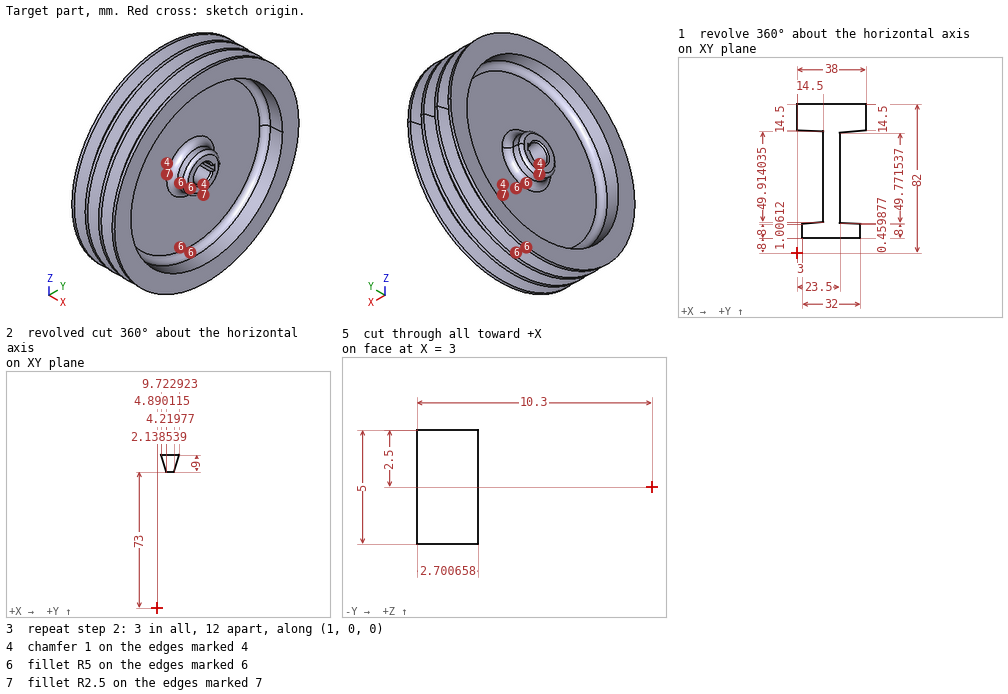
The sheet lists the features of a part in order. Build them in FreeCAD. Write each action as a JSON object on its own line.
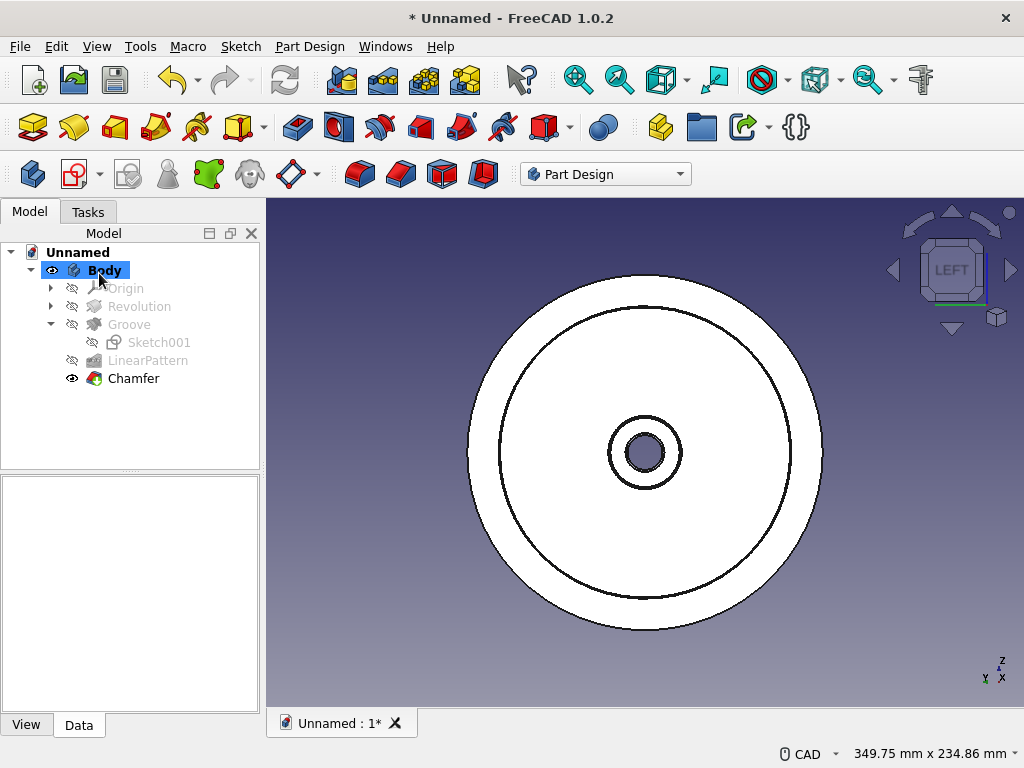
{"action": "scroll", "coordinate": [665, 471], "scroll_direction": "up", "scroll_amount": 3}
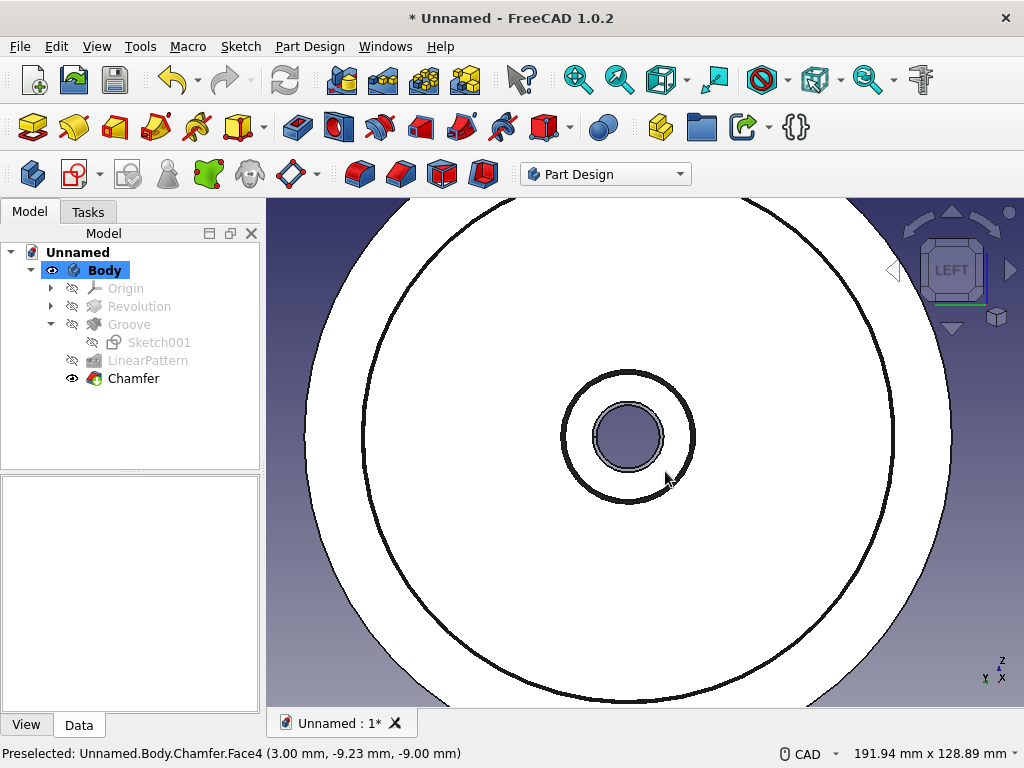
{"action": "left_click", "coordinate": [664, 472]}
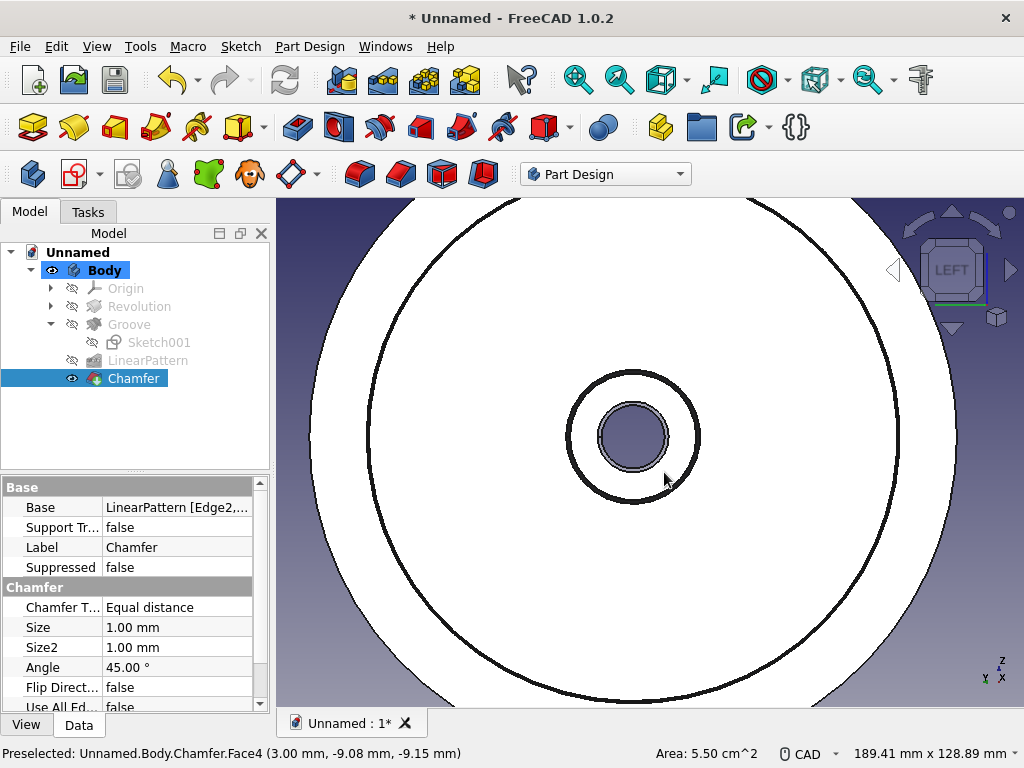
{"action": "left_click", "coordinate": [74, 174]}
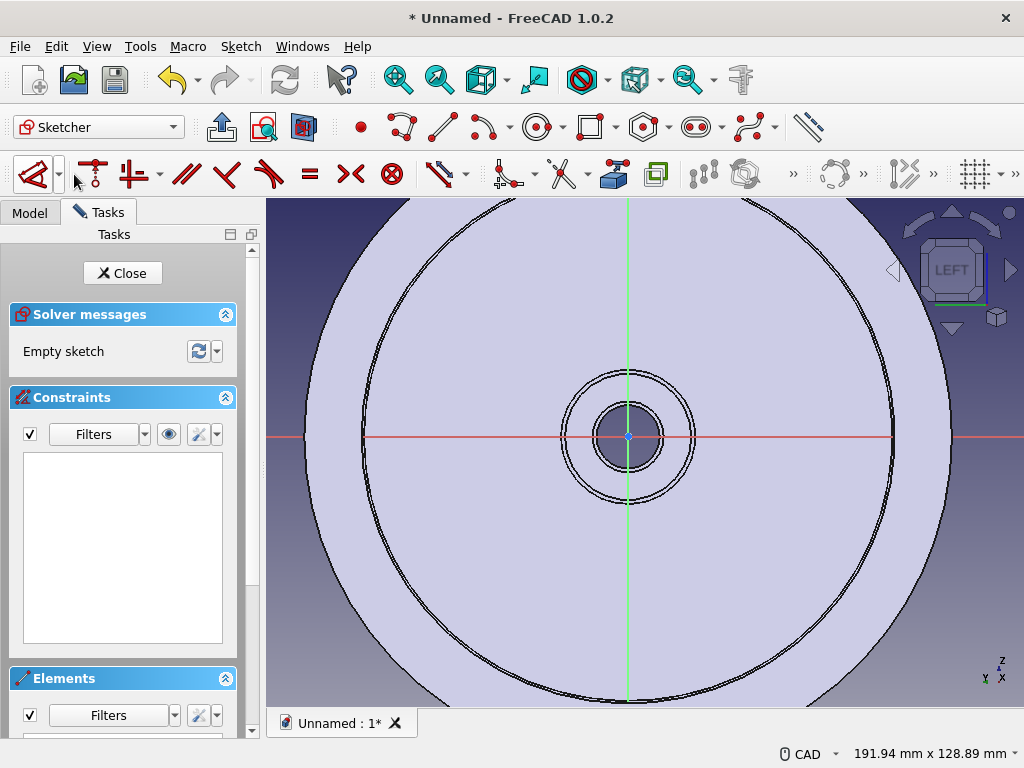
{"action": "left_click", "coordinate": [304, 128]}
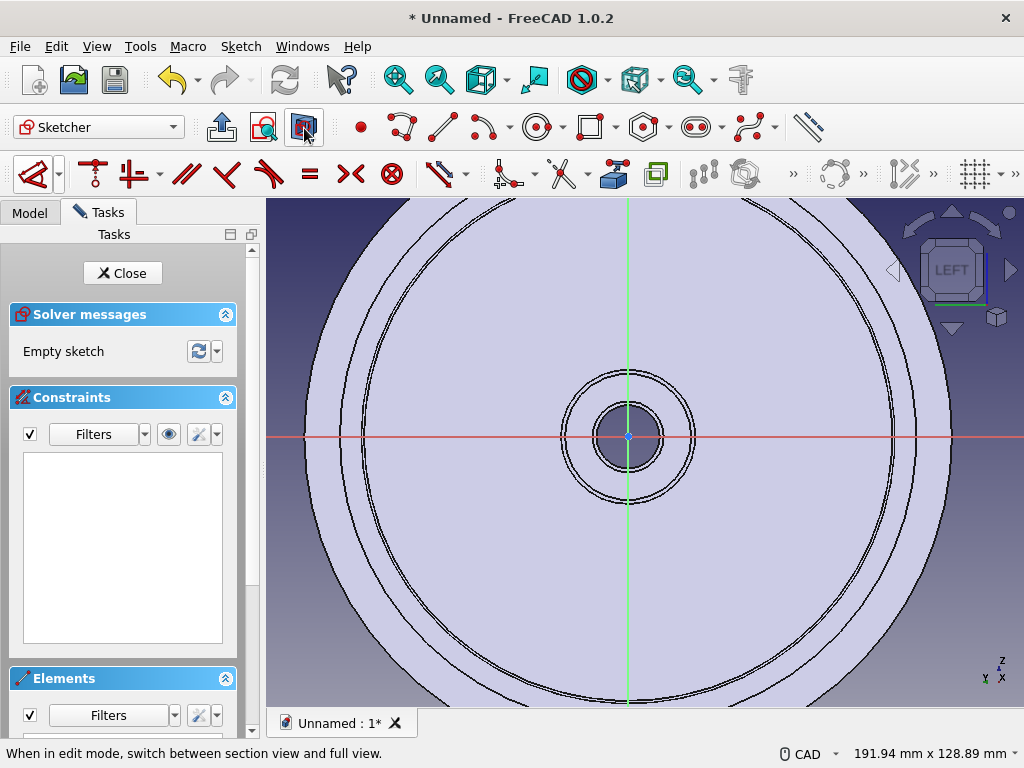
{"action": "scroll", "coordinate": [612, 435], "scroll_direction": "up", "scroll_amount": 11}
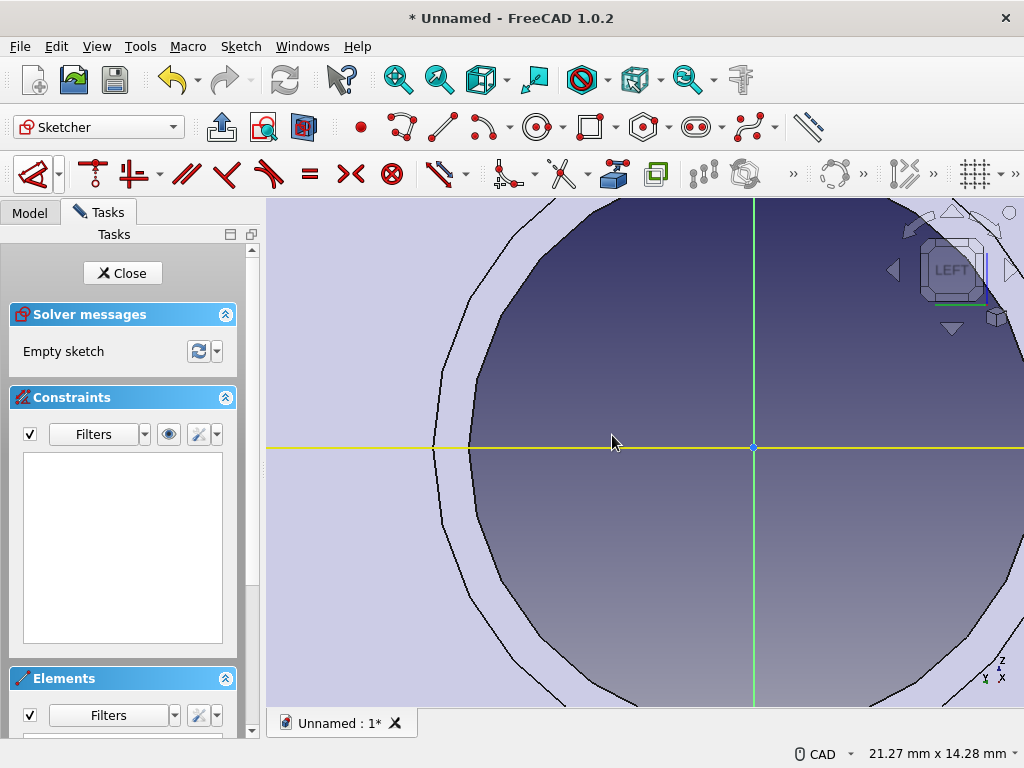
{"action": "left_click", "coordinate": [590, 128]}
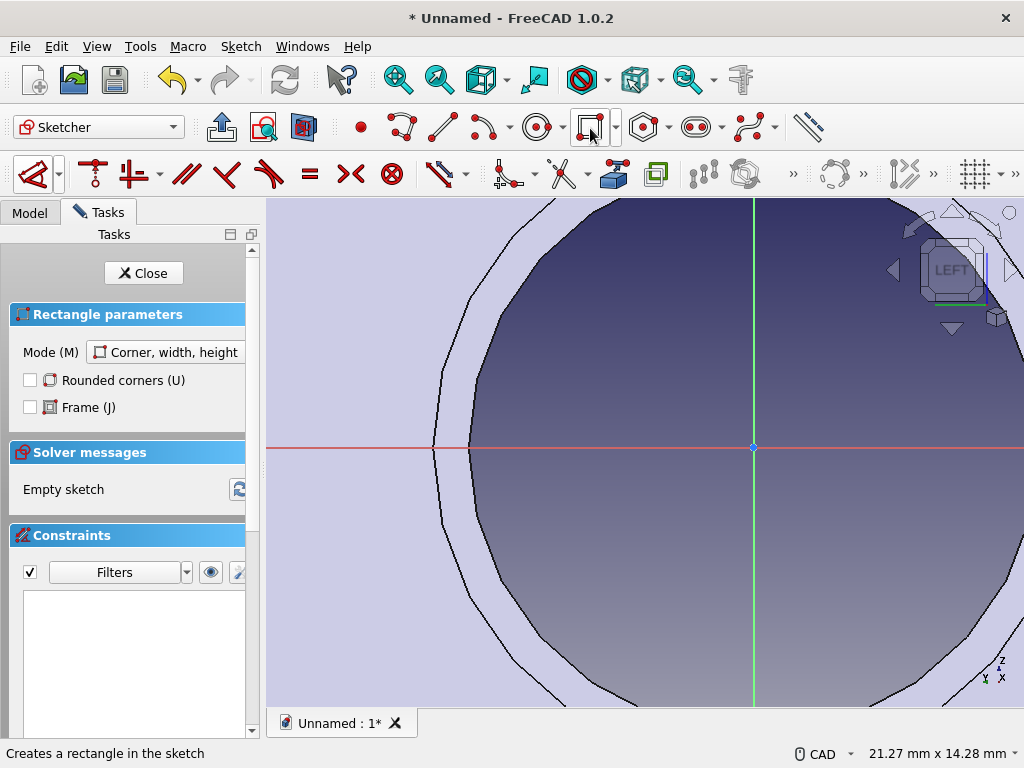
{"action": "left_click", "coordinate": [387, 359]}
{"action": "left_click", "coordinate": [483, 537]}
{"action": "key", "text": "Escape"}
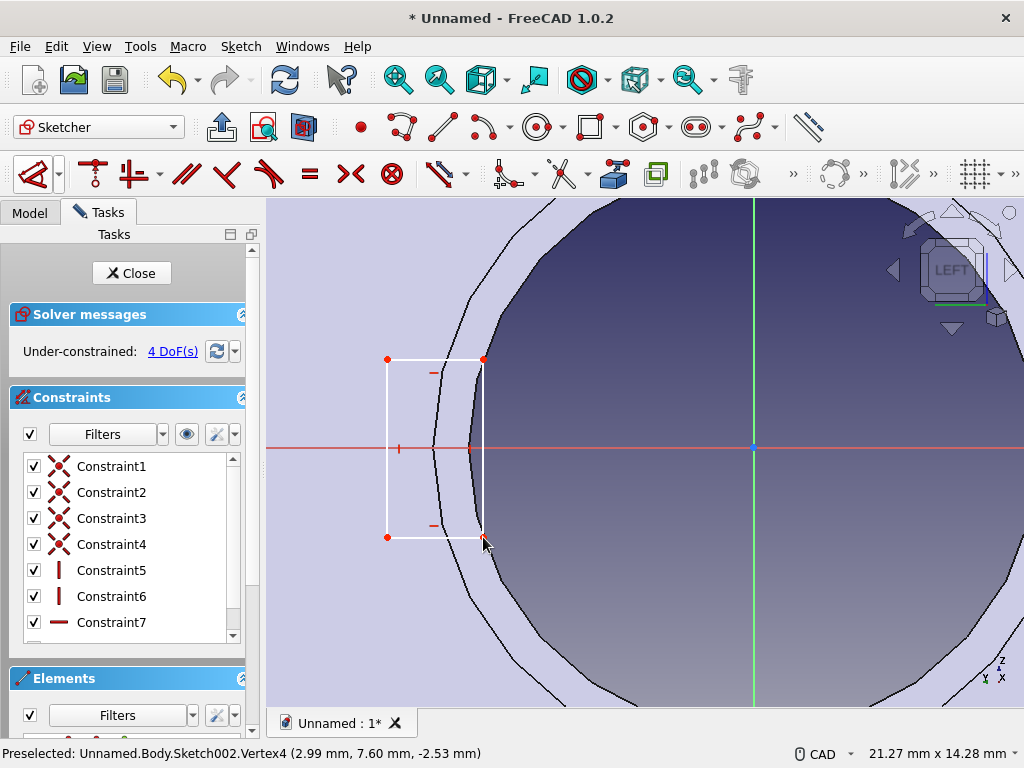
{"action": "left_click", "coordinate": [387, 413]}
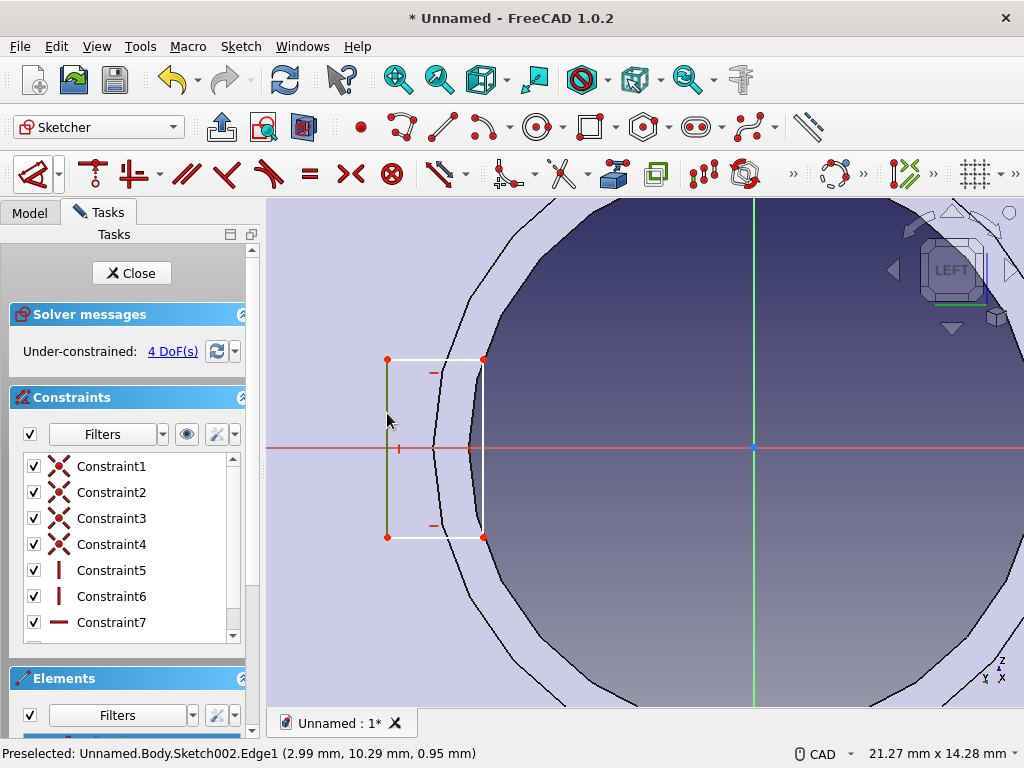
{"action": "left_click", "coordinate": [58, 174]}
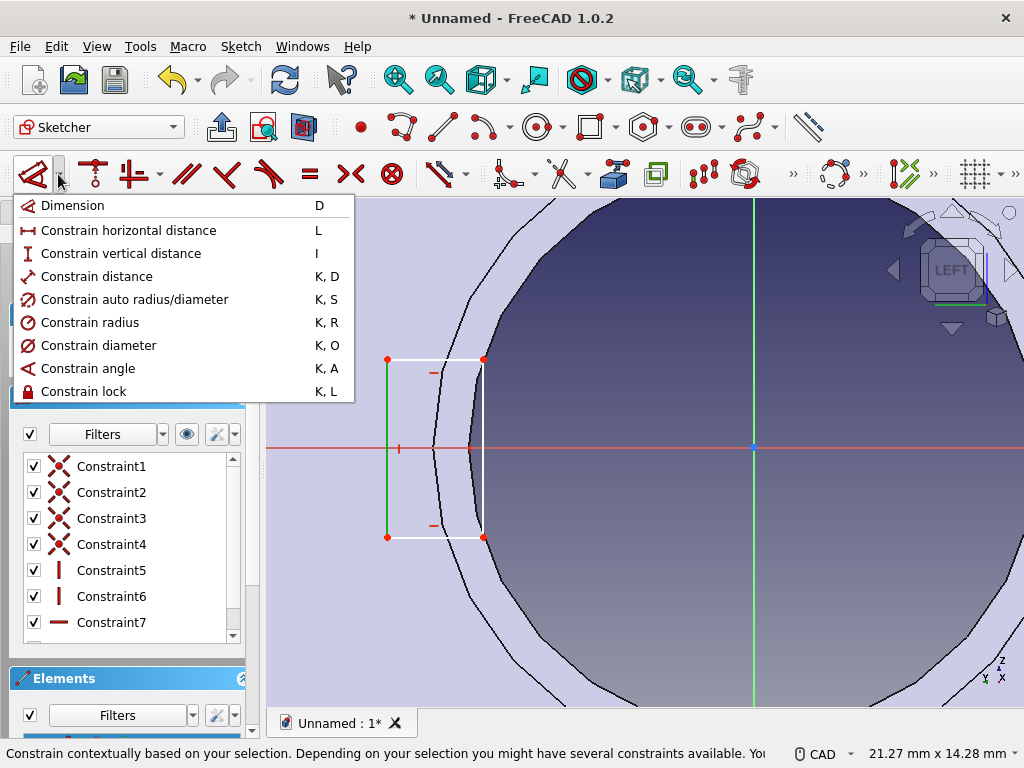
{"action": "left_click", "coordinate": [184, 254]}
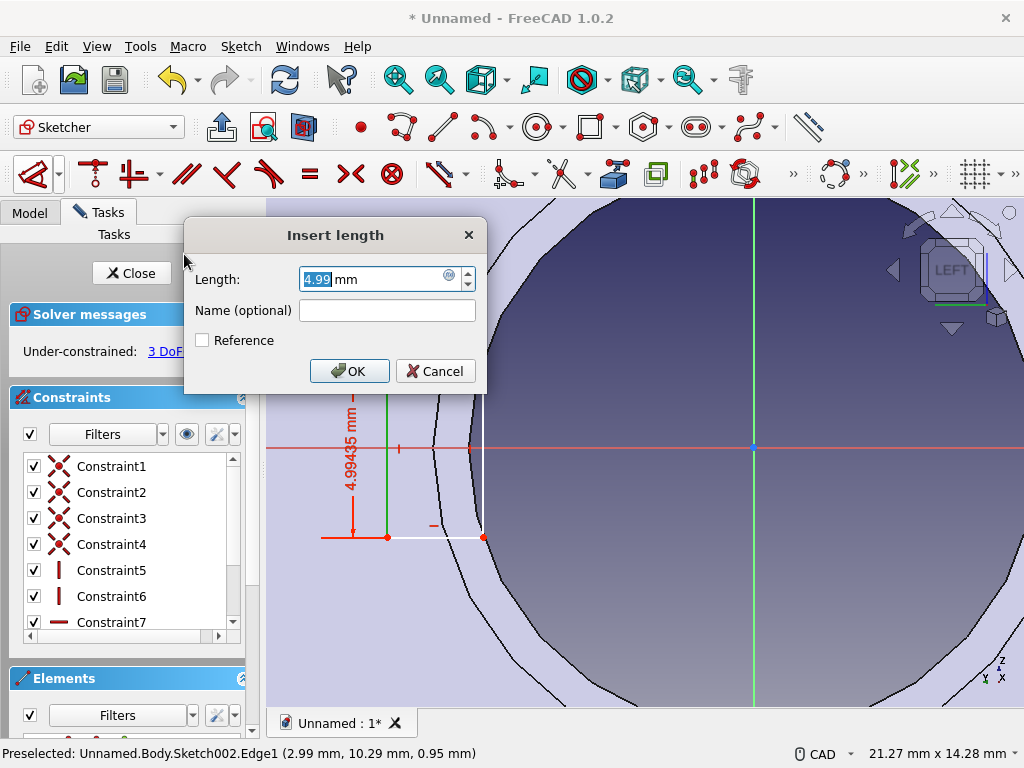
{"action": "type", "text": "5"}
{"action": "key", "text": "Return"}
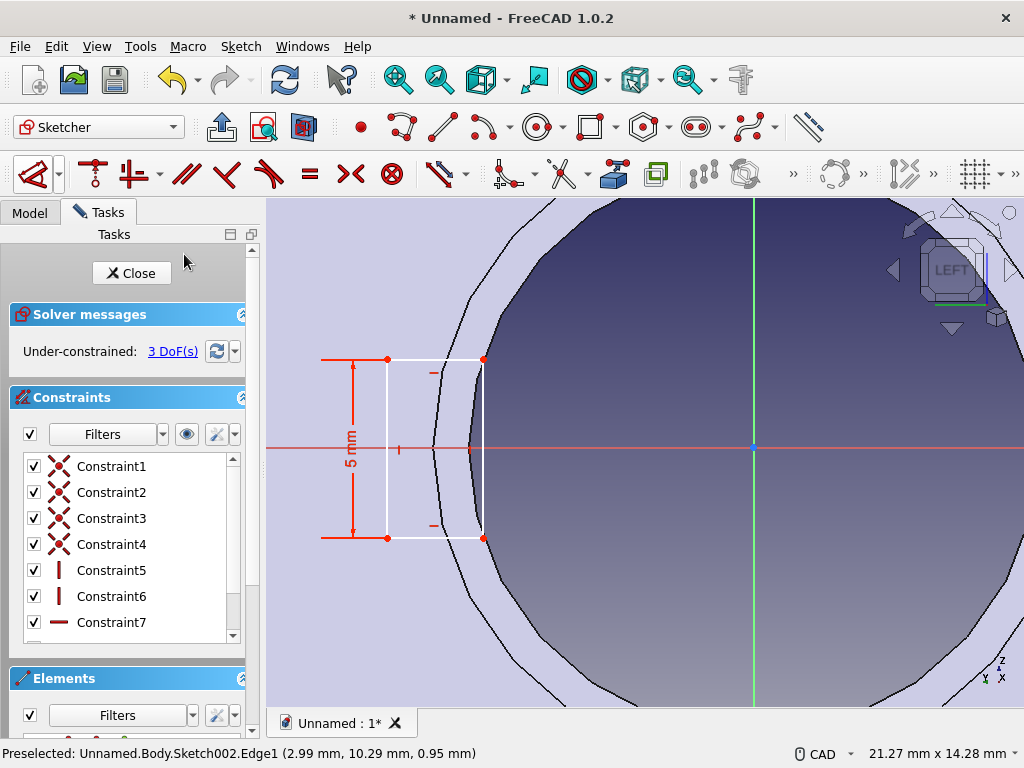
{"action": "left_click", "coordinate": [387, 360]}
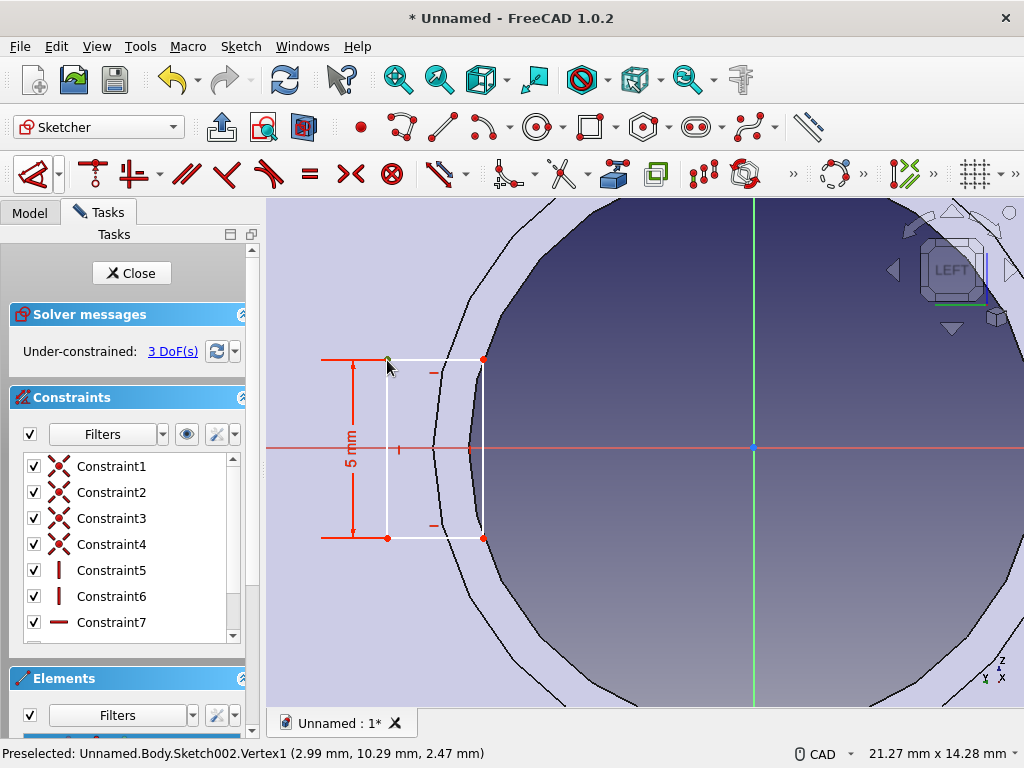
{"action": "key", "text": "i"}